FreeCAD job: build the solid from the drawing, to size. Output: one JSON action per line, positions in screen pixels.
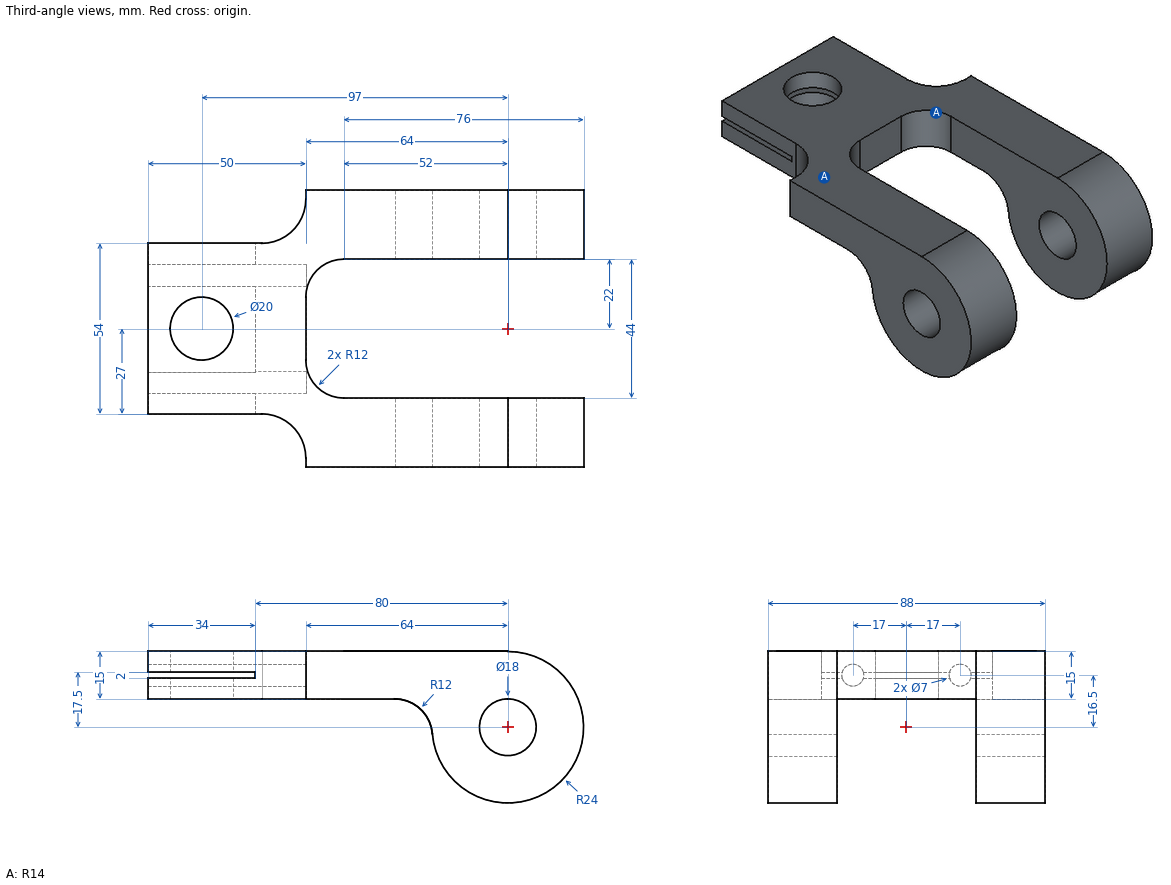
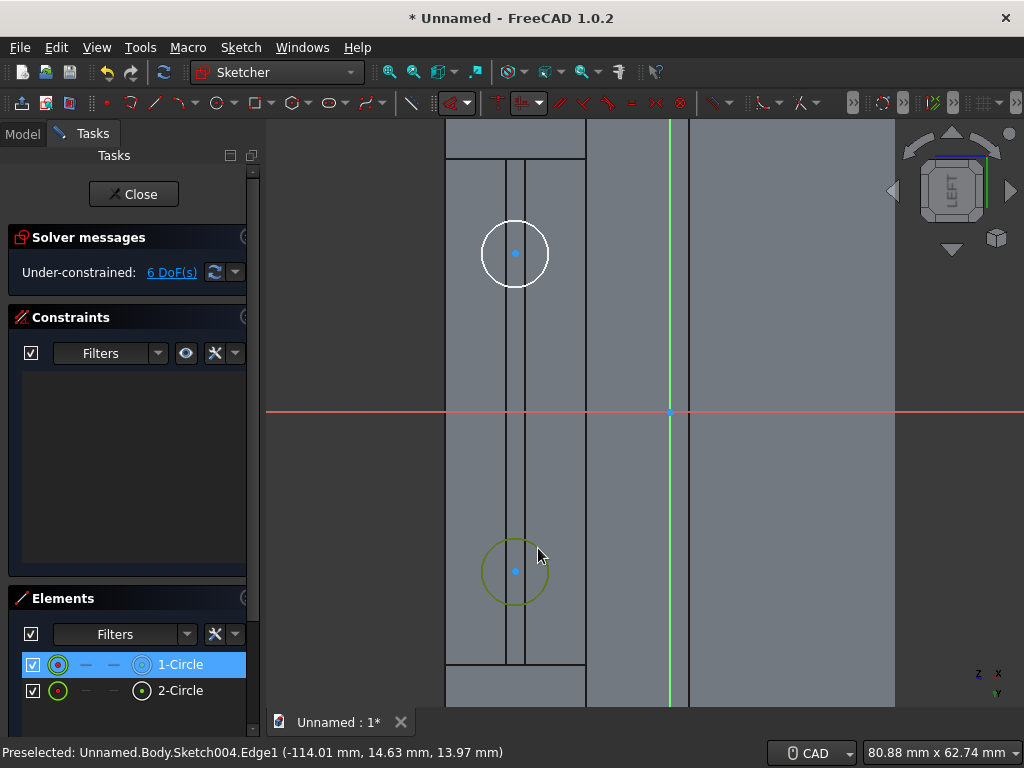
{"action": "left_click", "coordinate": [538, 230]}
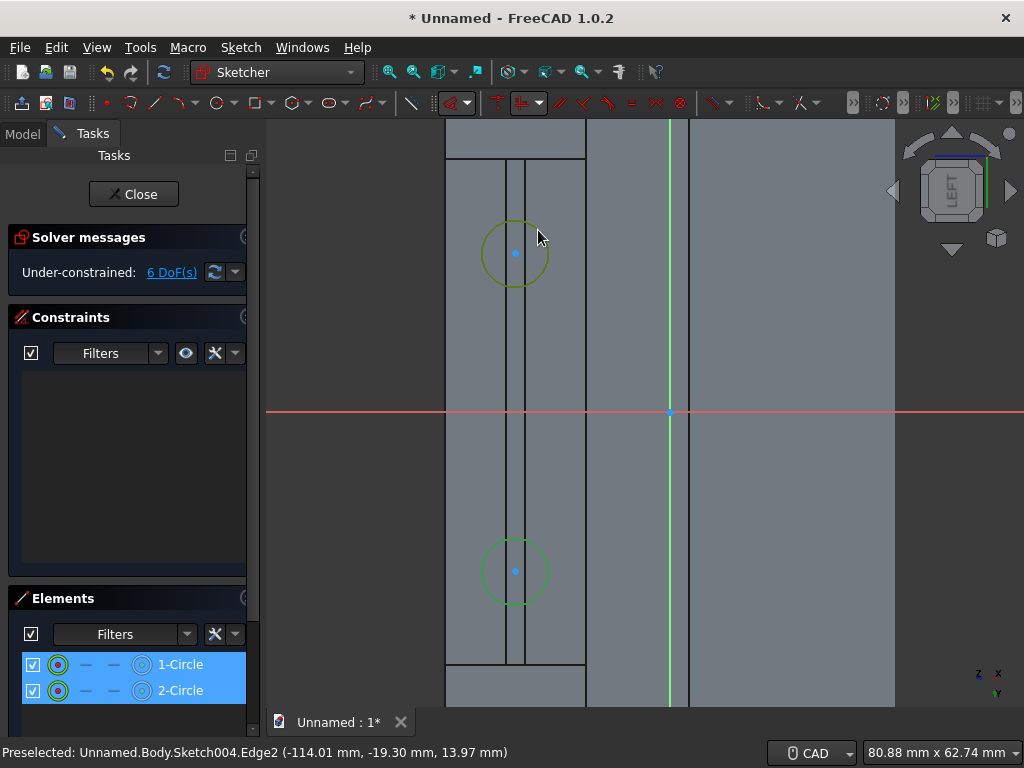
{"action": "left_click", "coordinate": [632, 104]}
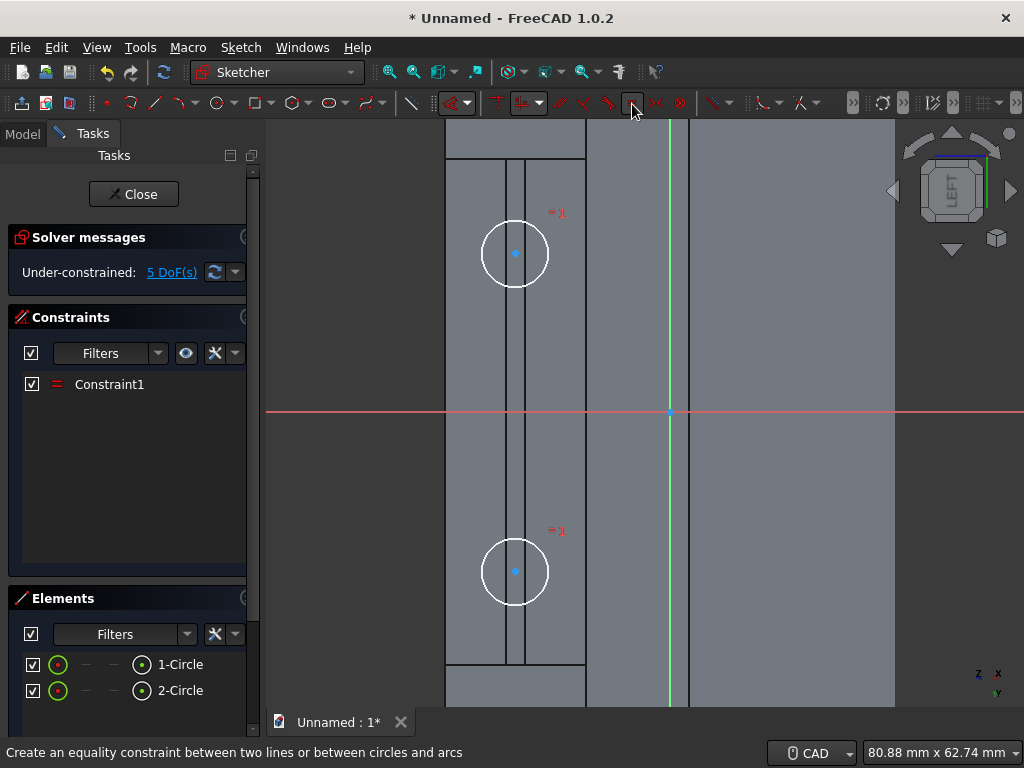
{"action": "left_click", "coordinate": [515, 572]}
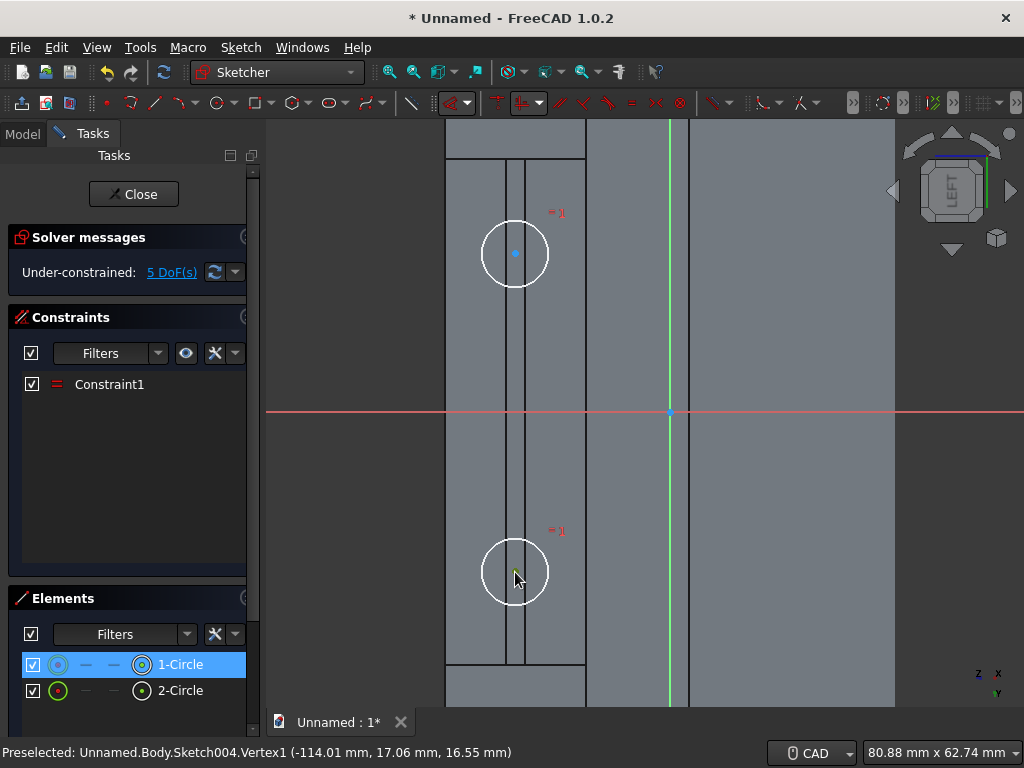
{"action": "left_click", "coordinate": [515, 254]}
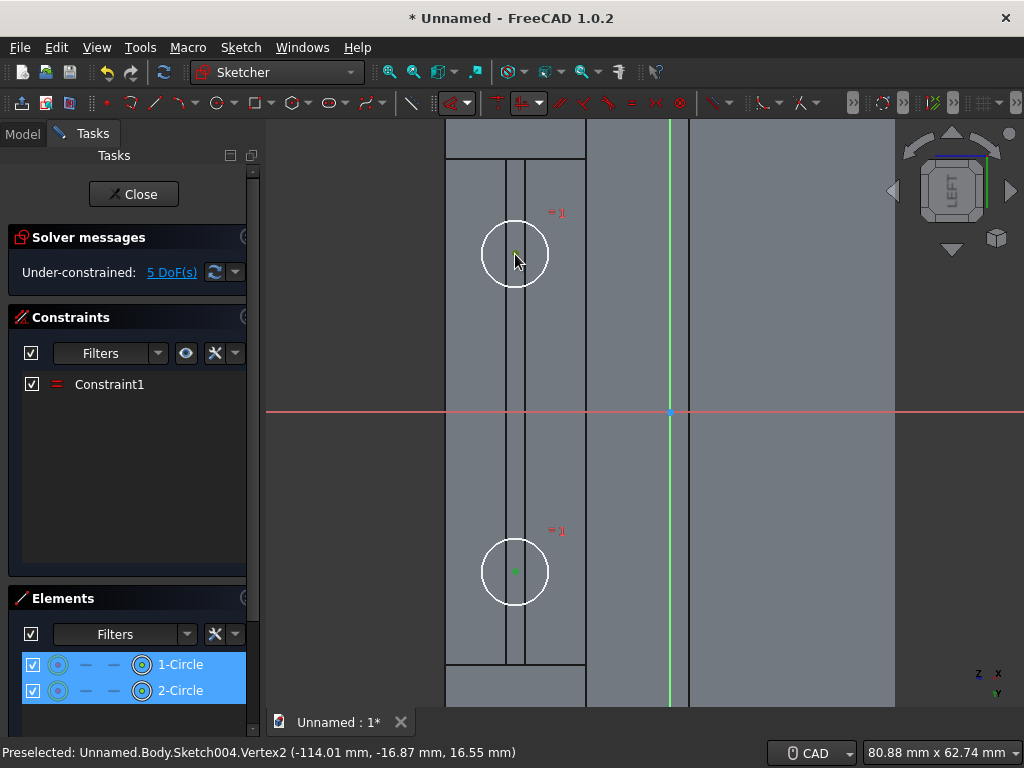
{"action": "left_click", "coordinate": [542, 104]}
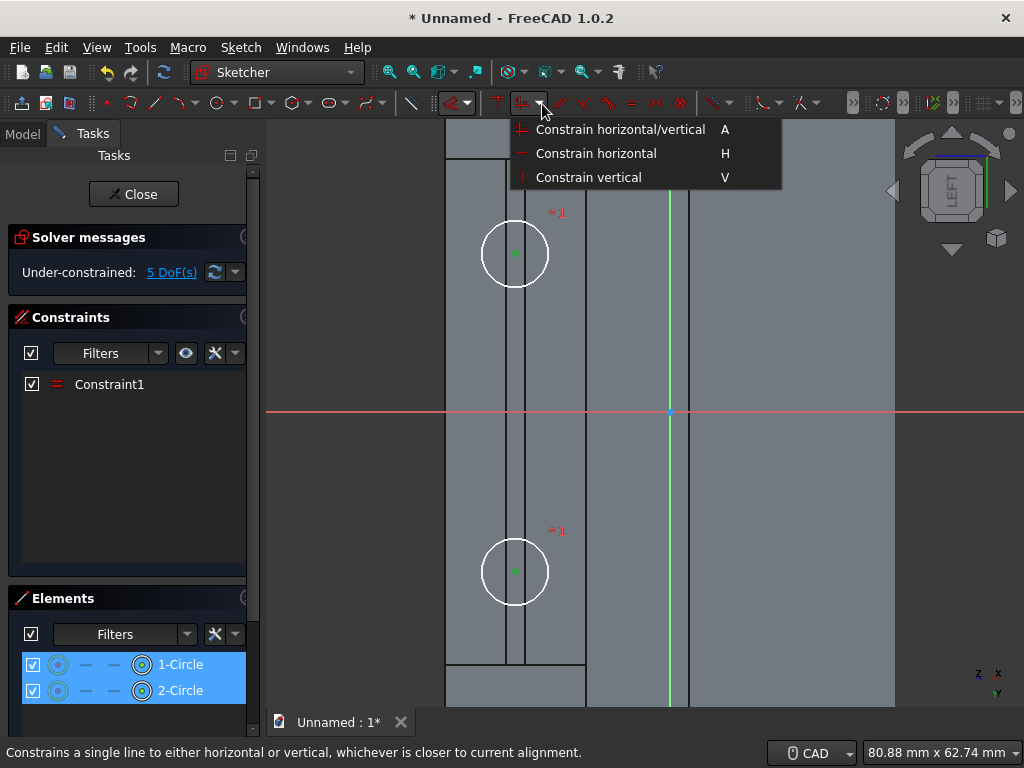
{"action": "left_click", "coordinate": [646, 177]}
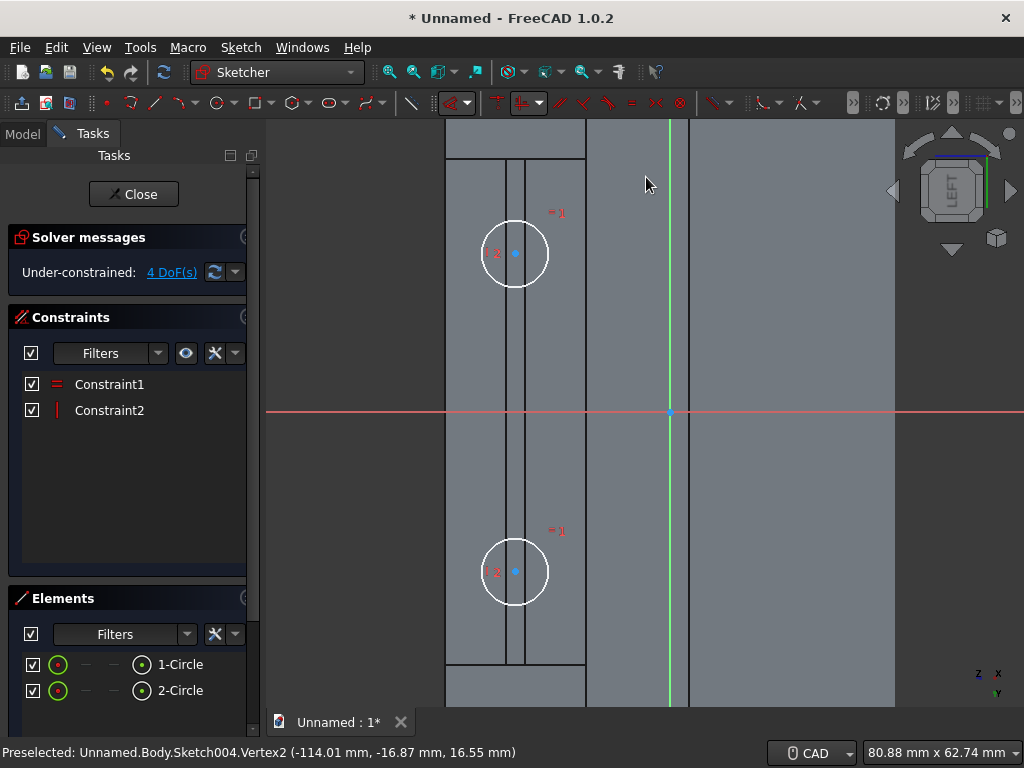
{"action": "left_click", "coordinate": [538, 548]}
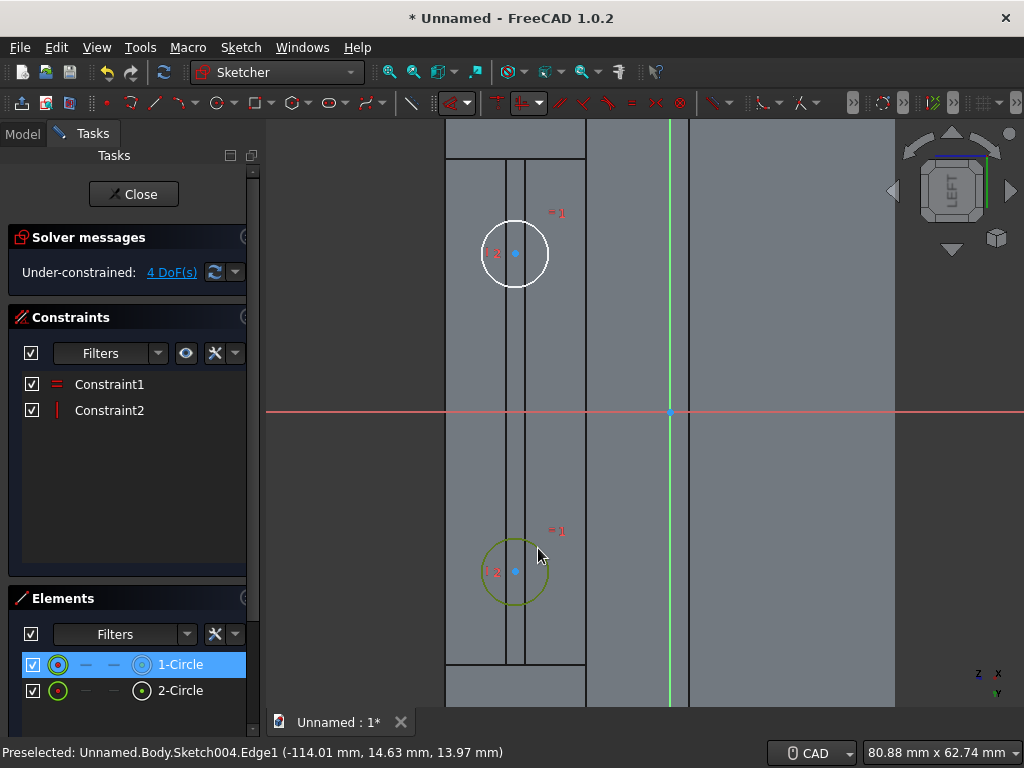
{"action": "left_click", "coordinate": [470, 104]}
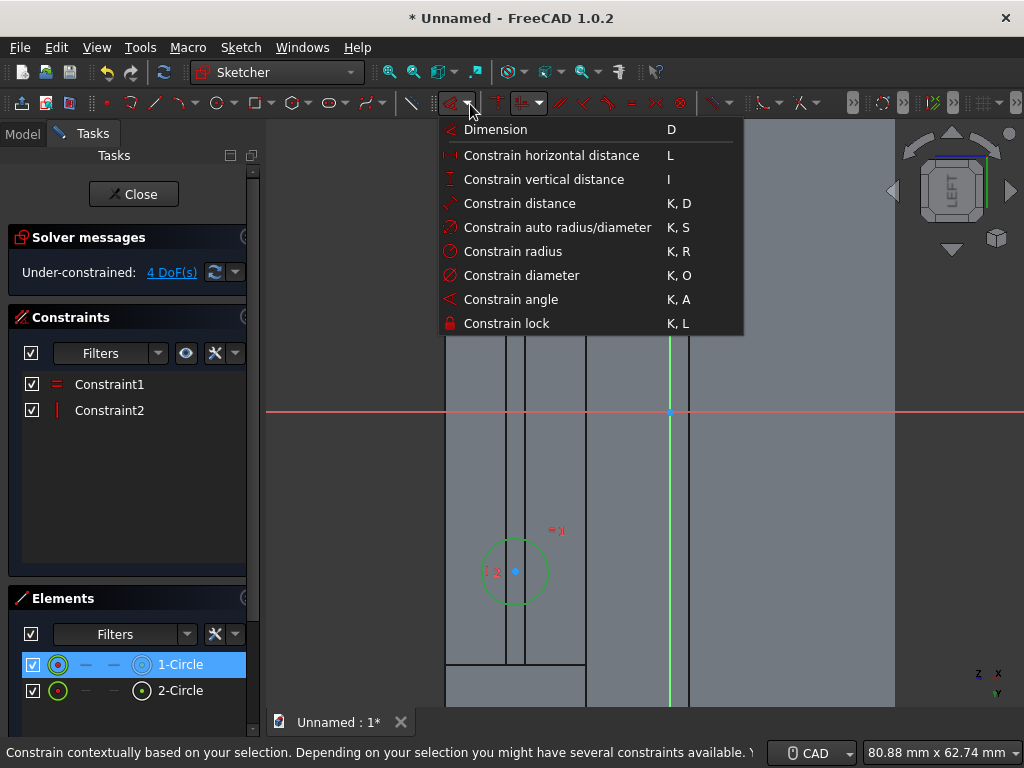
{"action": "left_click", "coordinate": [591, 275]}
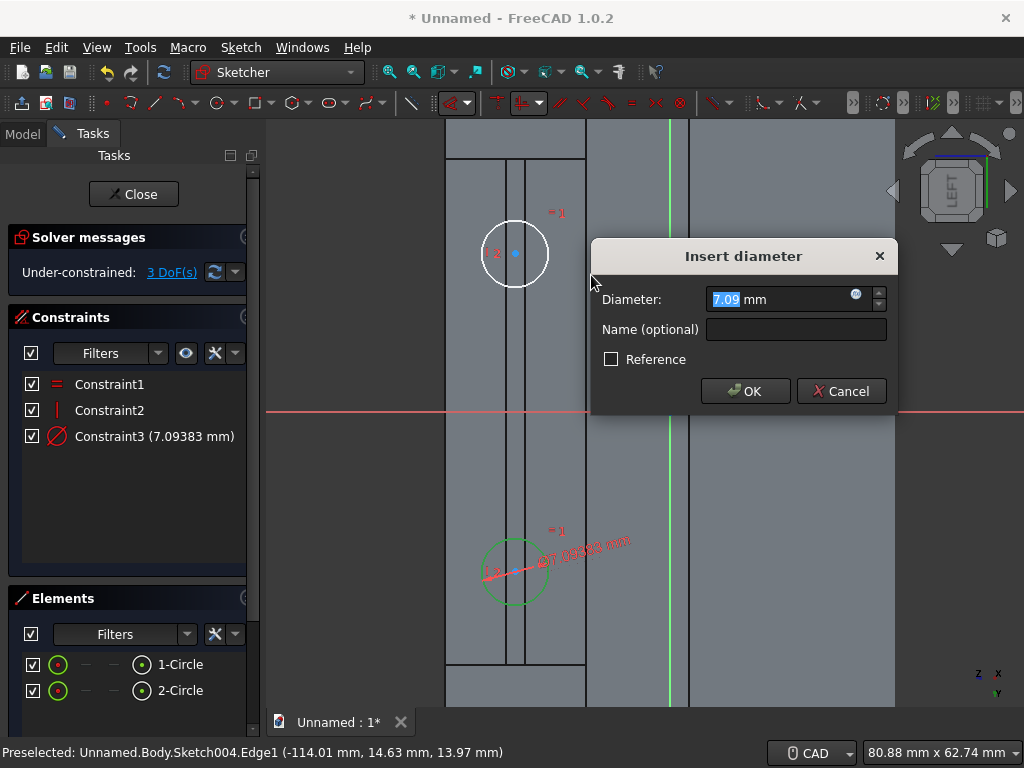
{"action": "type", "text": "7"}
{"action": "key", "text": "Return"}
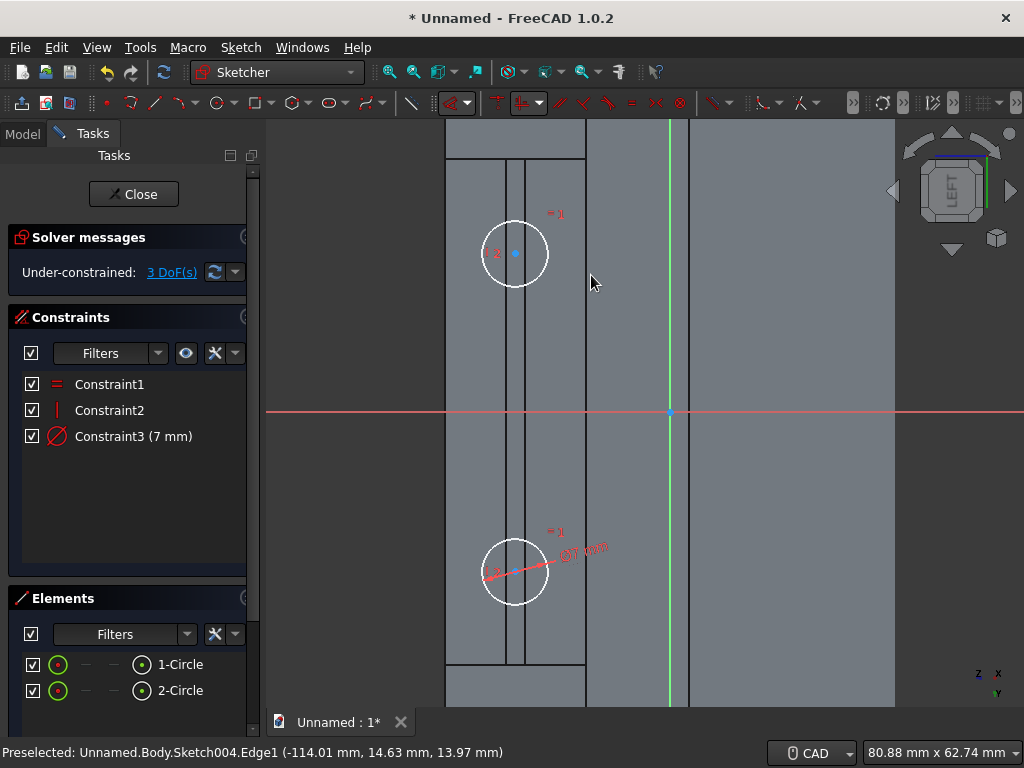
{"action": "left_click", "coordinate": [515, 572]}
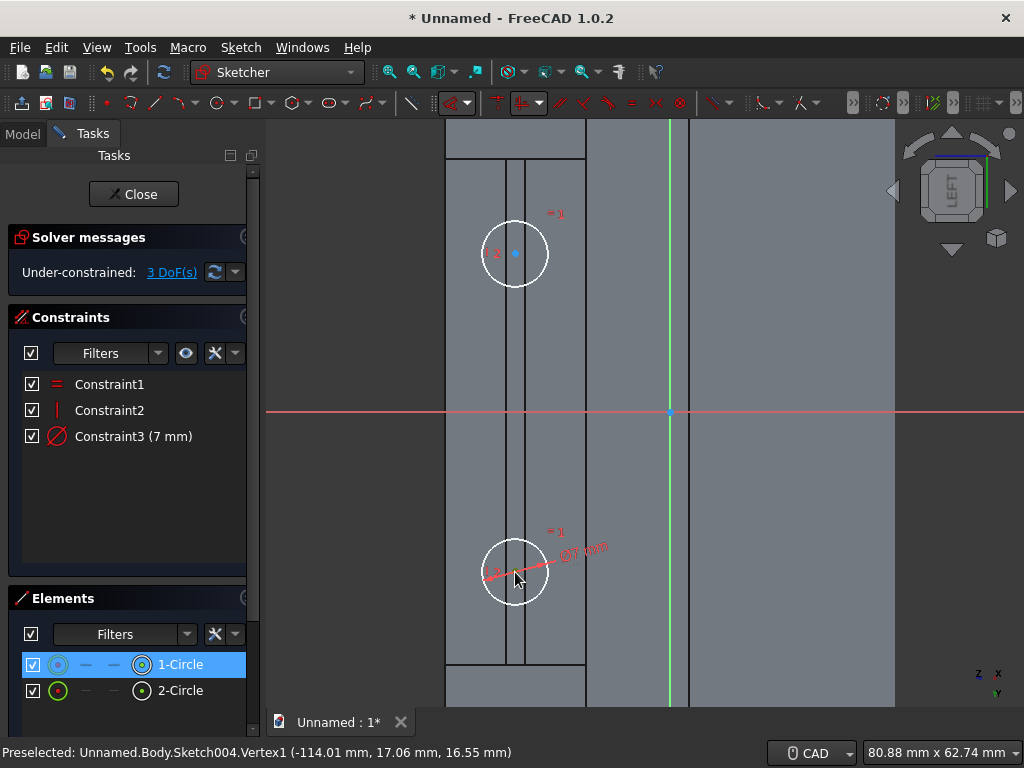
{"action": "key", "text": "i"}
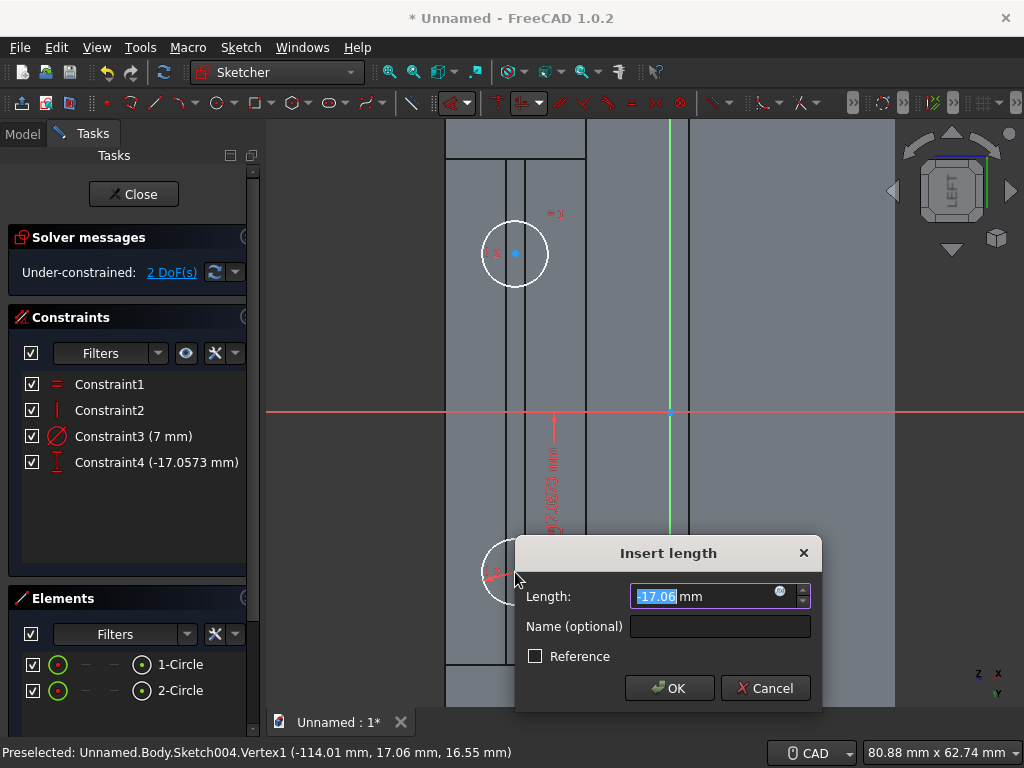
{"action": "type", "text": "-17"}
{"action": "key", "text": "Return"}